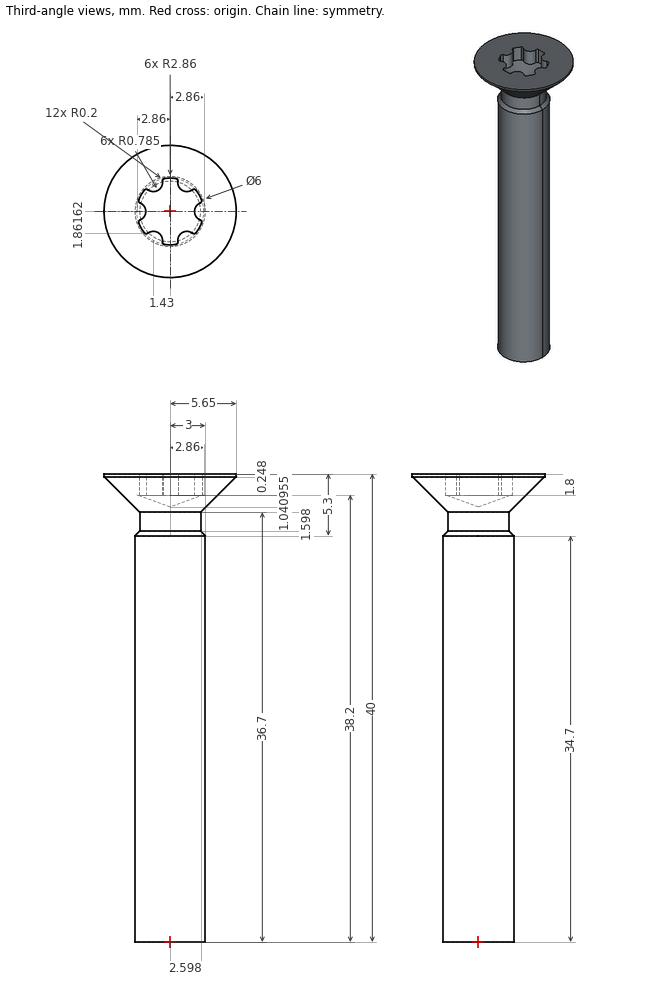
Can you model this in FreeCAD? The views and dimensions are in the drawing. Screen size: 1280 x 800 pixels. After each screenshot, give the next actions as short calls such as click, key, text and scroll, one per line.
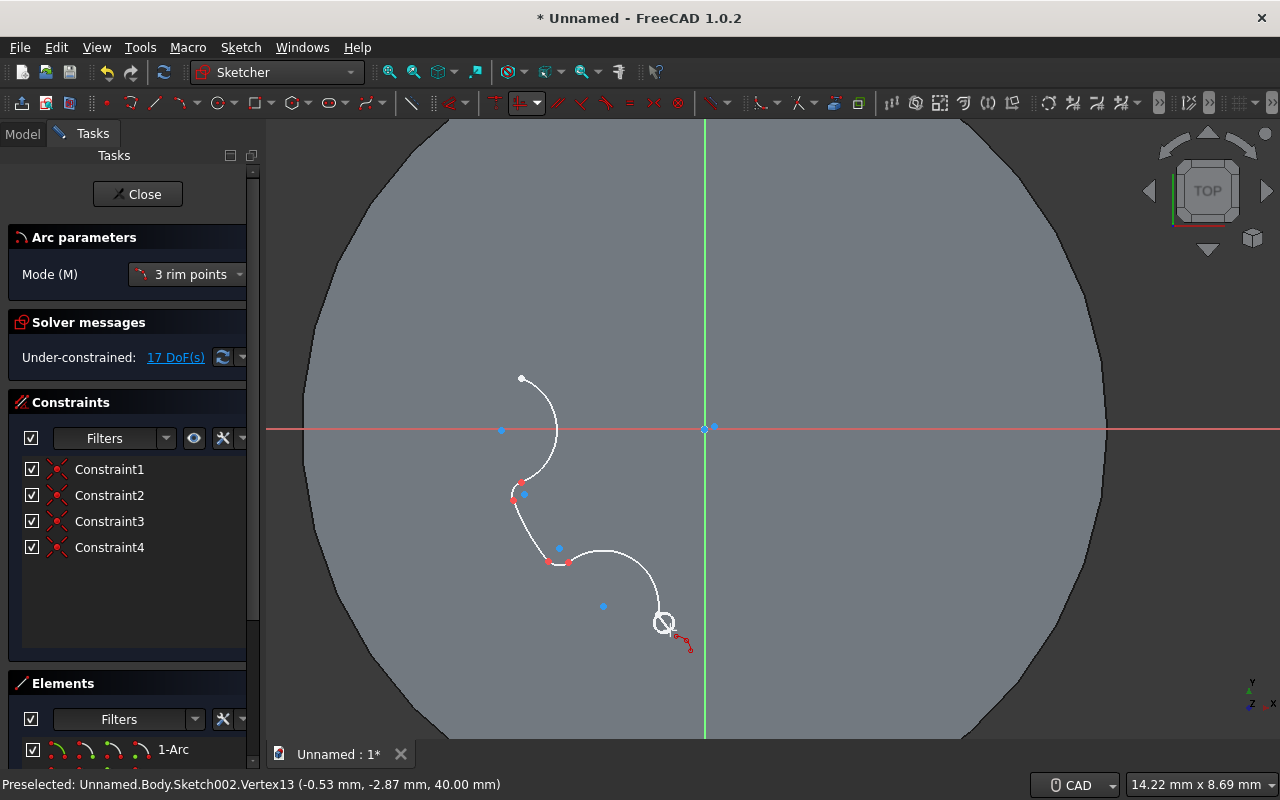
scroll(660, 625, up, 7)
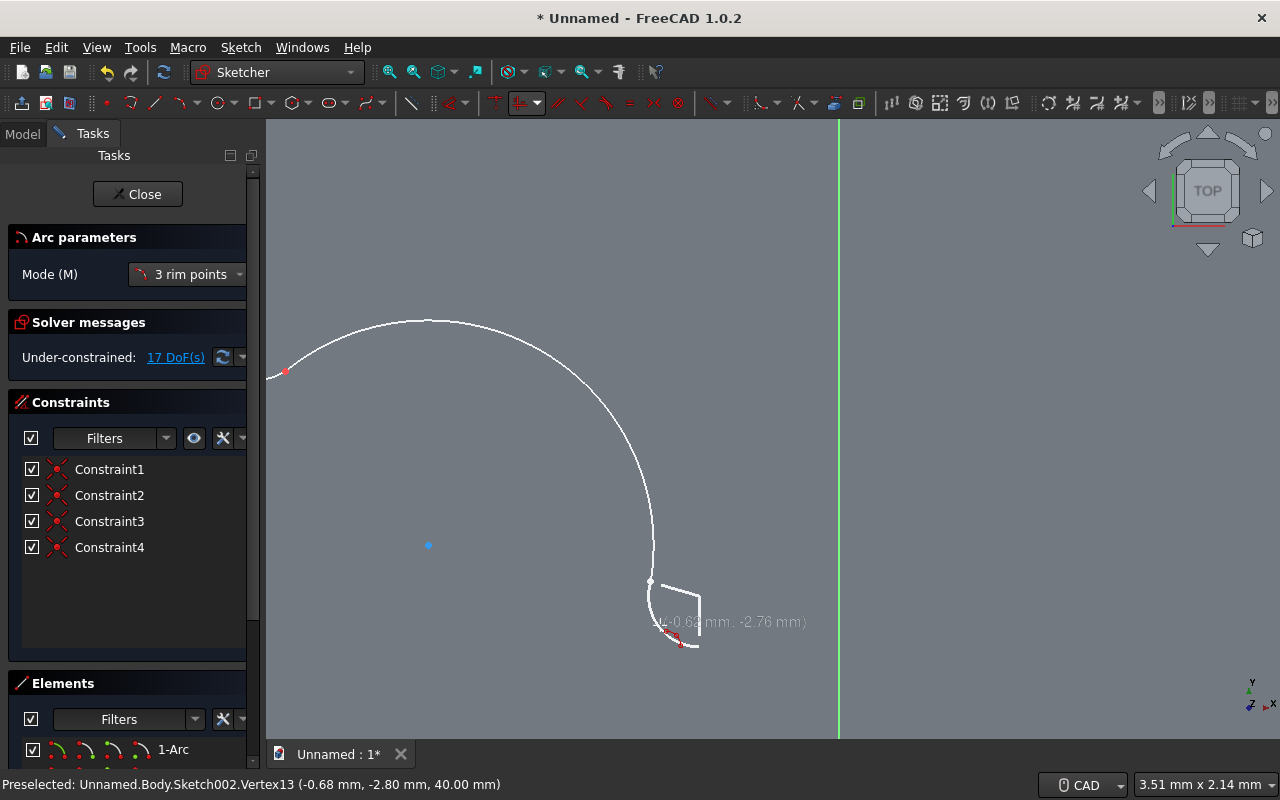
click(661, 621)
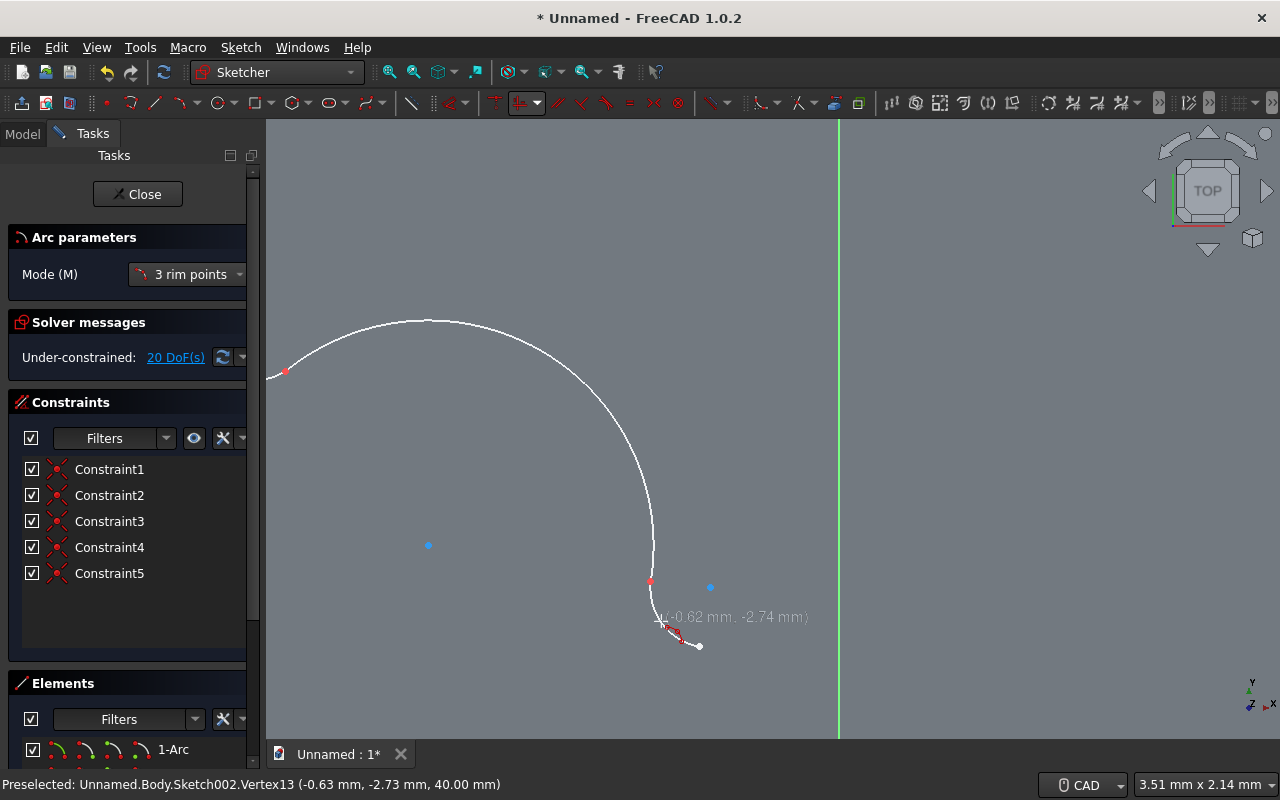
scroll(660, 625, down, 7)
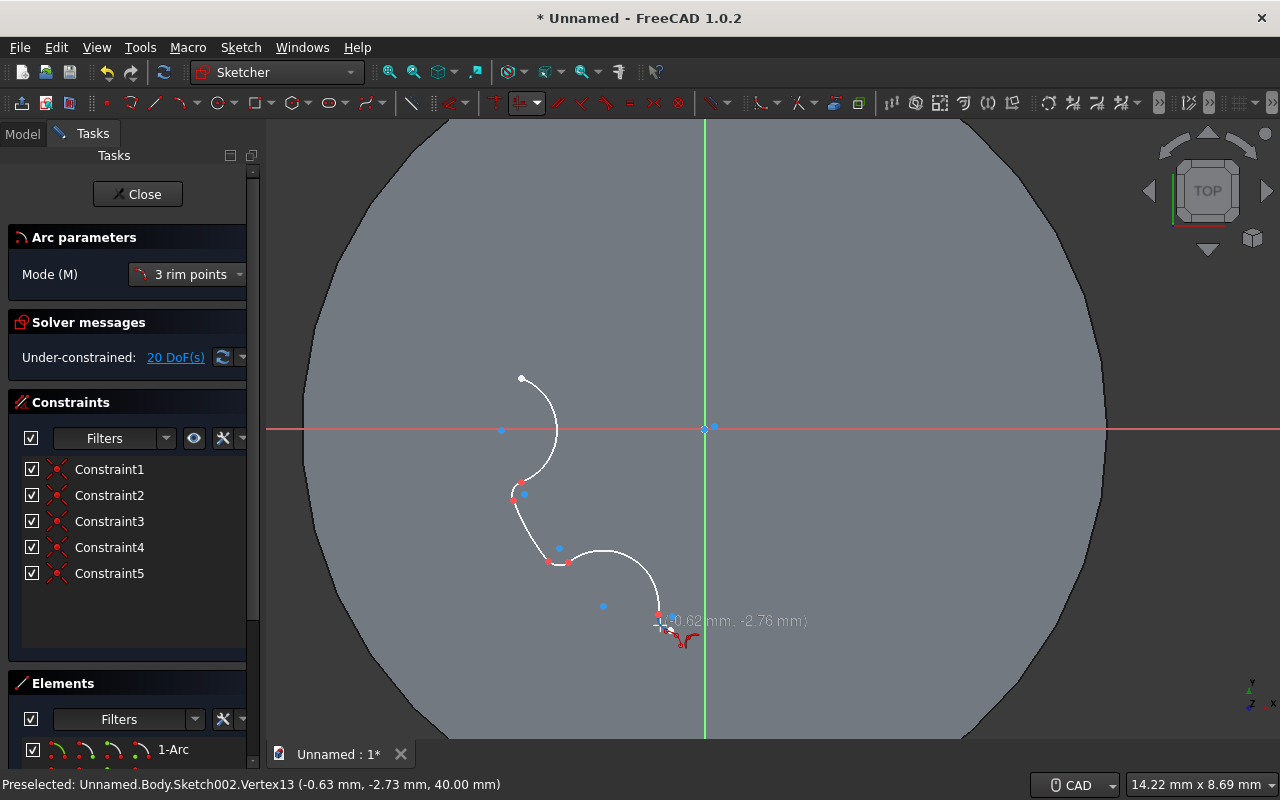
click(670, 631)
click(739, 630)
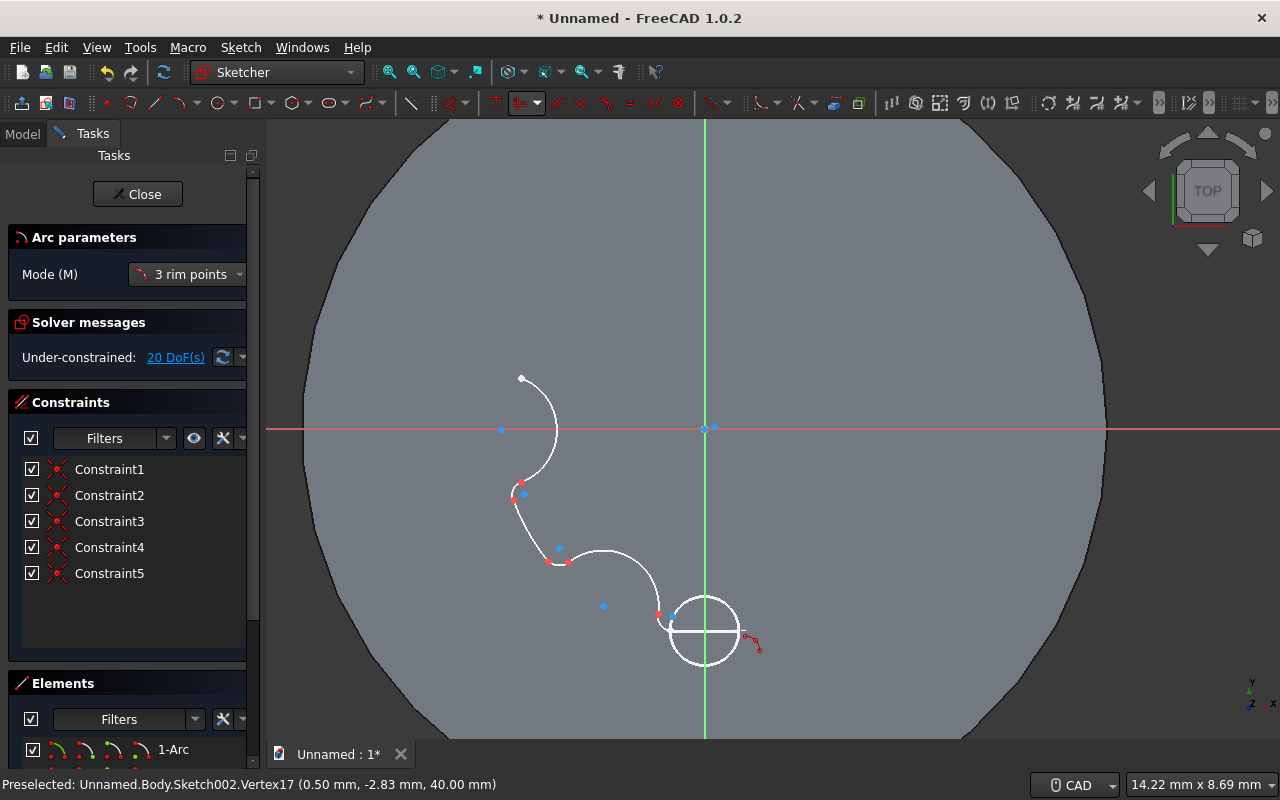
scroll(698, 633, up, 9)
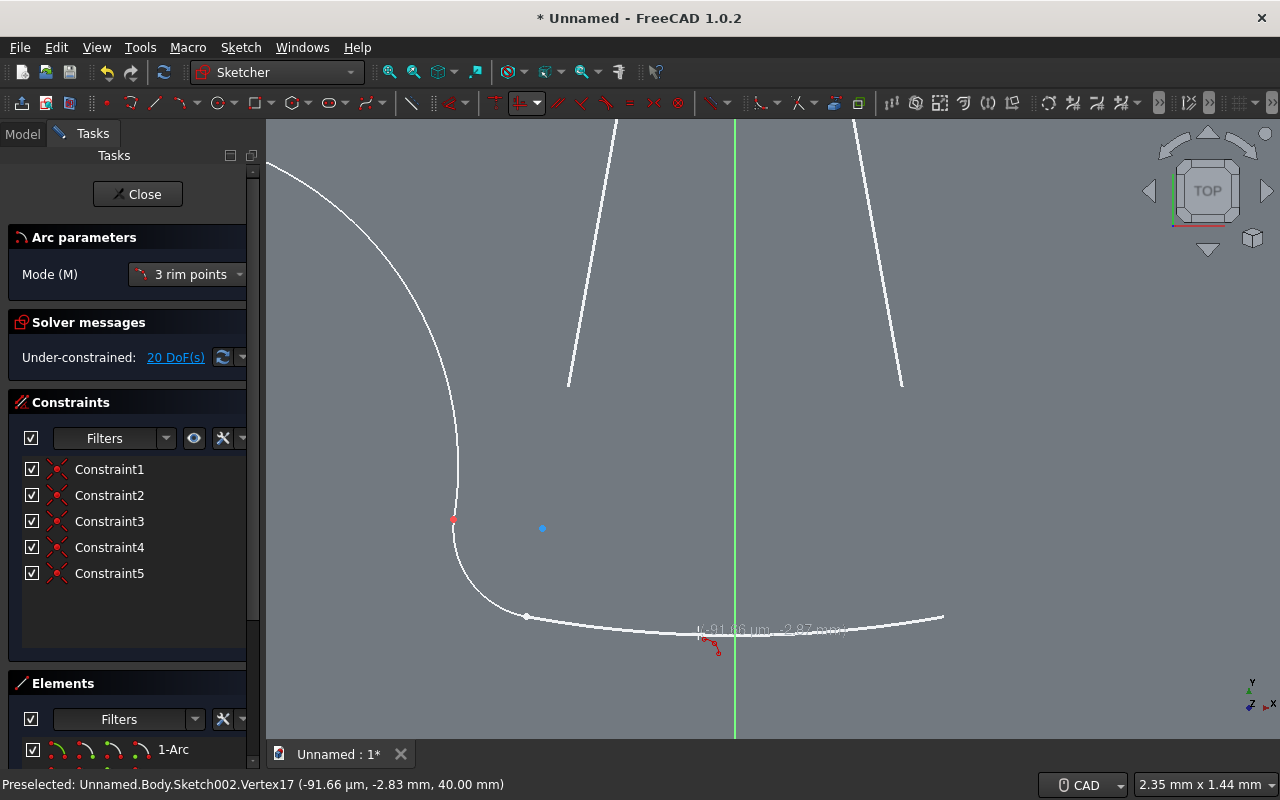
click(693, 629)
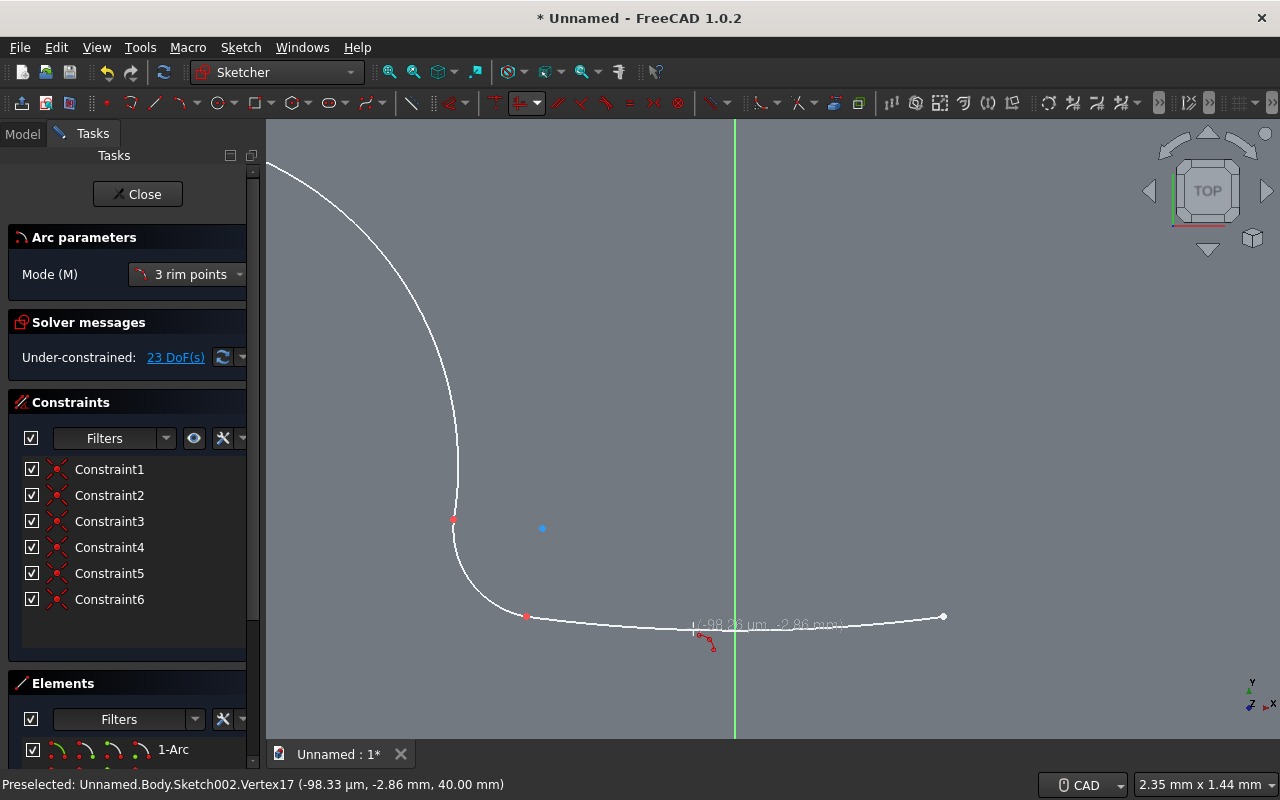
scroll(698, 633, down, 9)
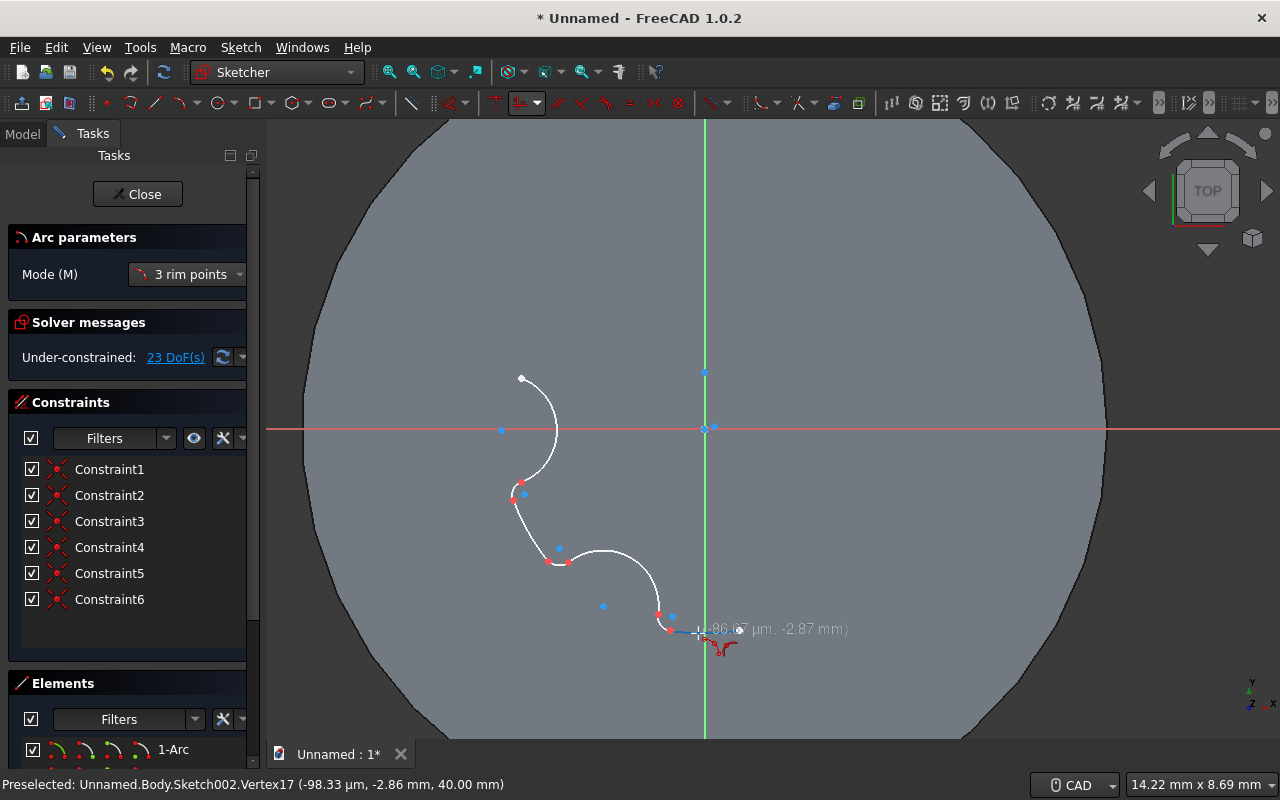
click(739, 631)
click(751, 614)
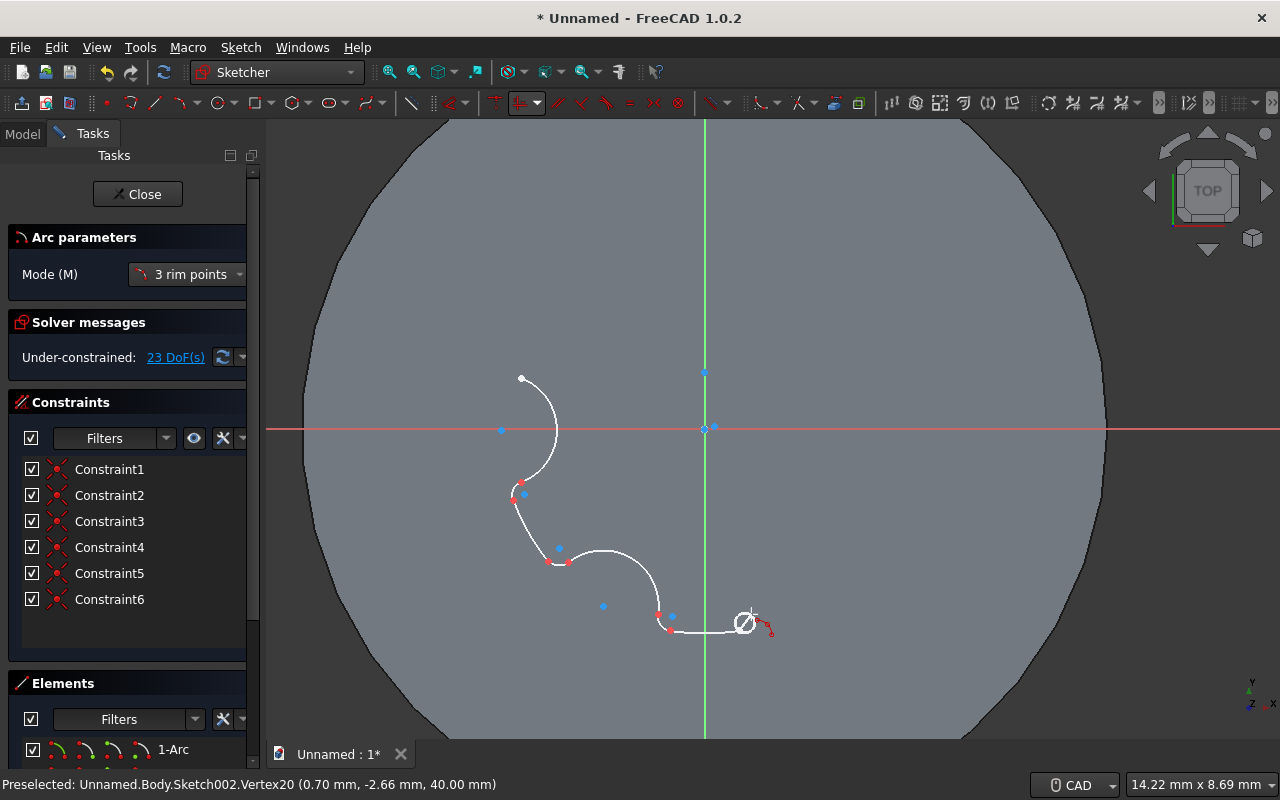
scroll(749, 625, up, 7)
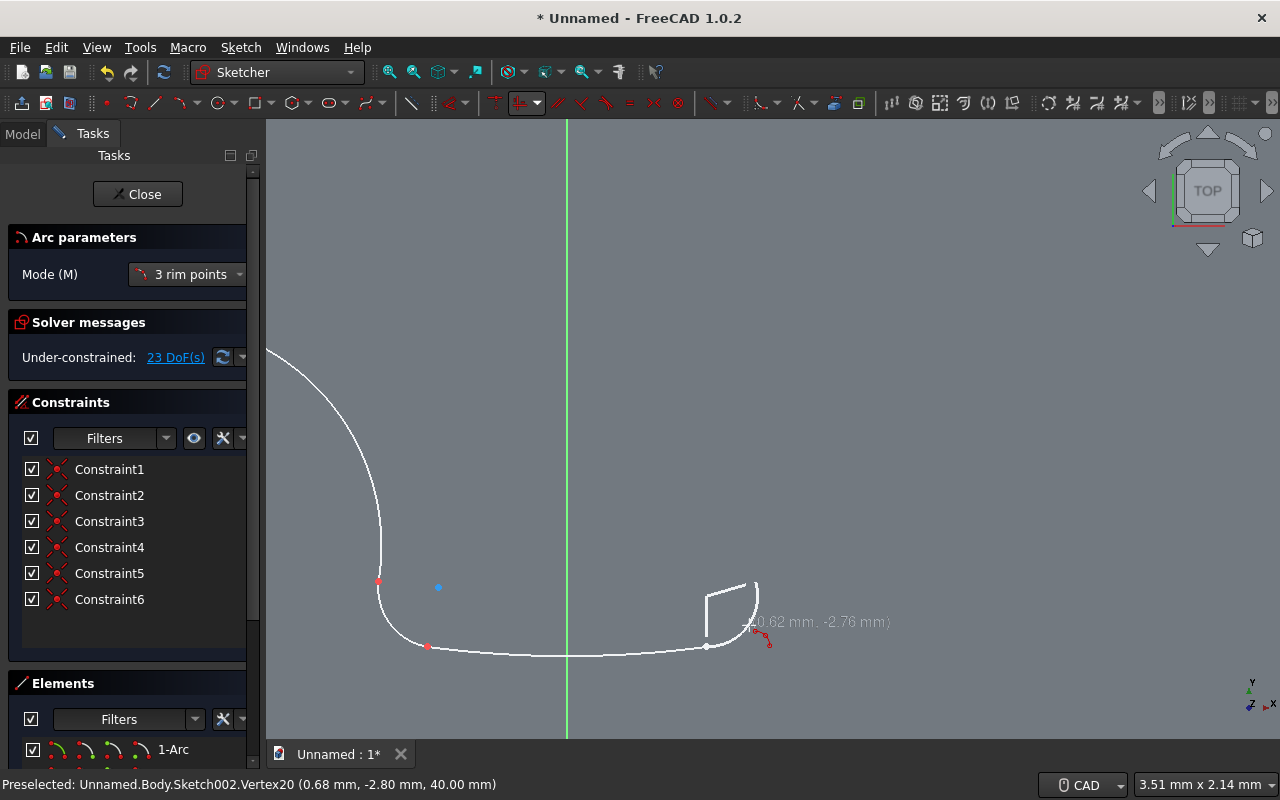
click(746, 621)